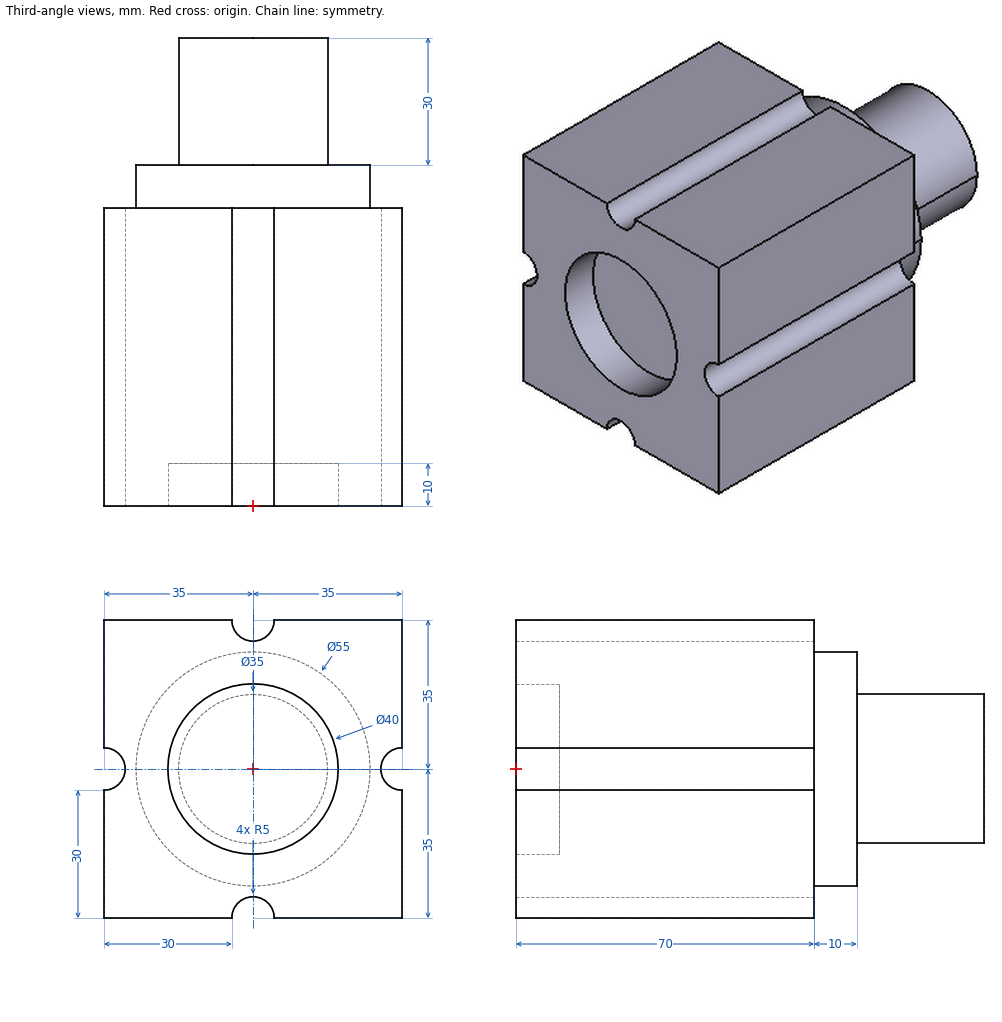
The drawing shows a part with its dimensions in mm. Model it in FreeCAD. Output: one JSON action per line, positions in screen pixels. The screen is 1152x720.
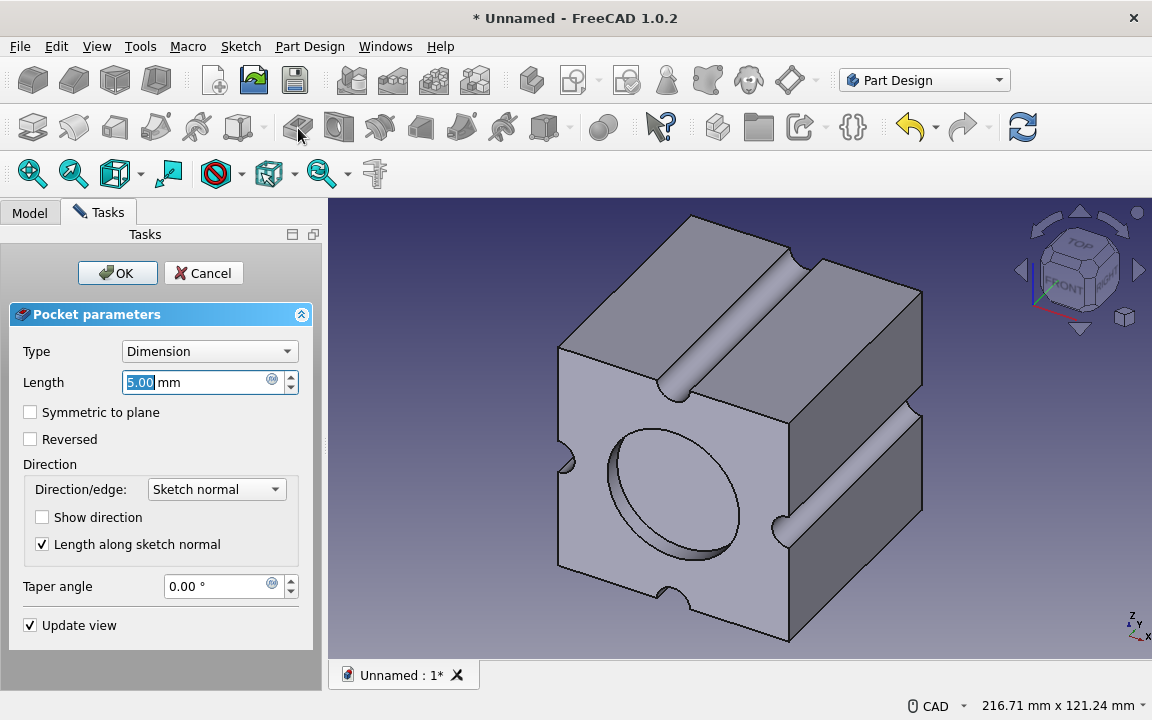
{"action": "type", "text": "10"}
{"action": "key", "text": "Tab"}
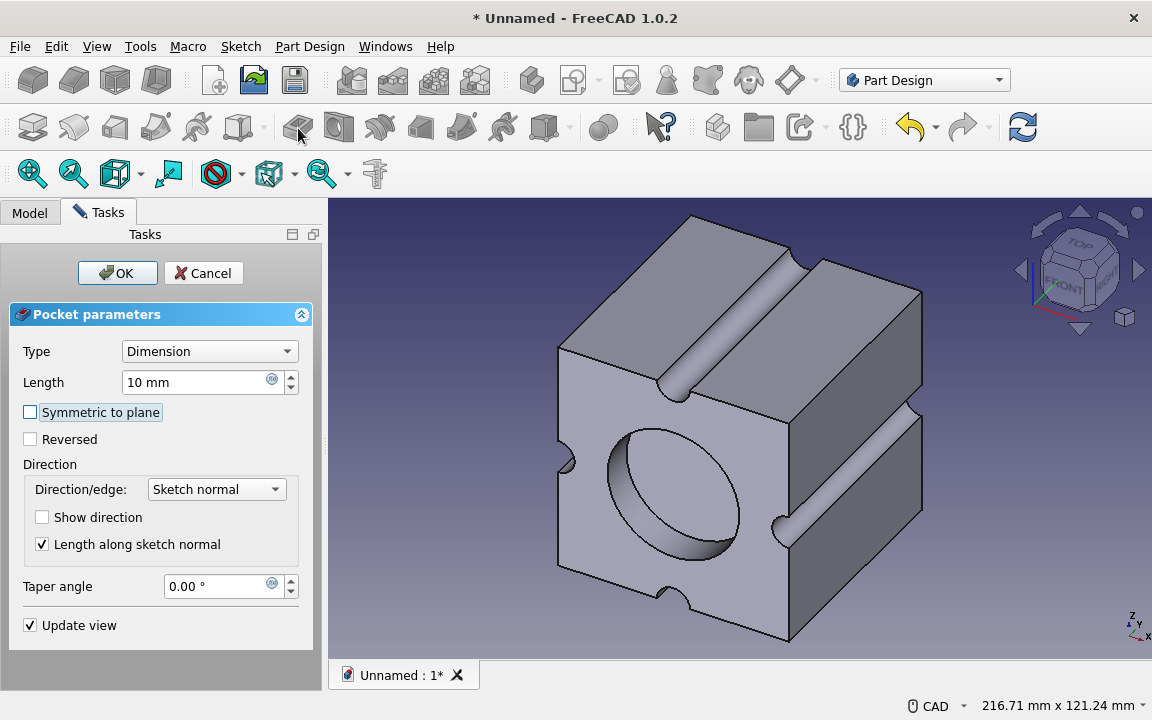
{"action": "left_click", "coordinate": [118, 273]}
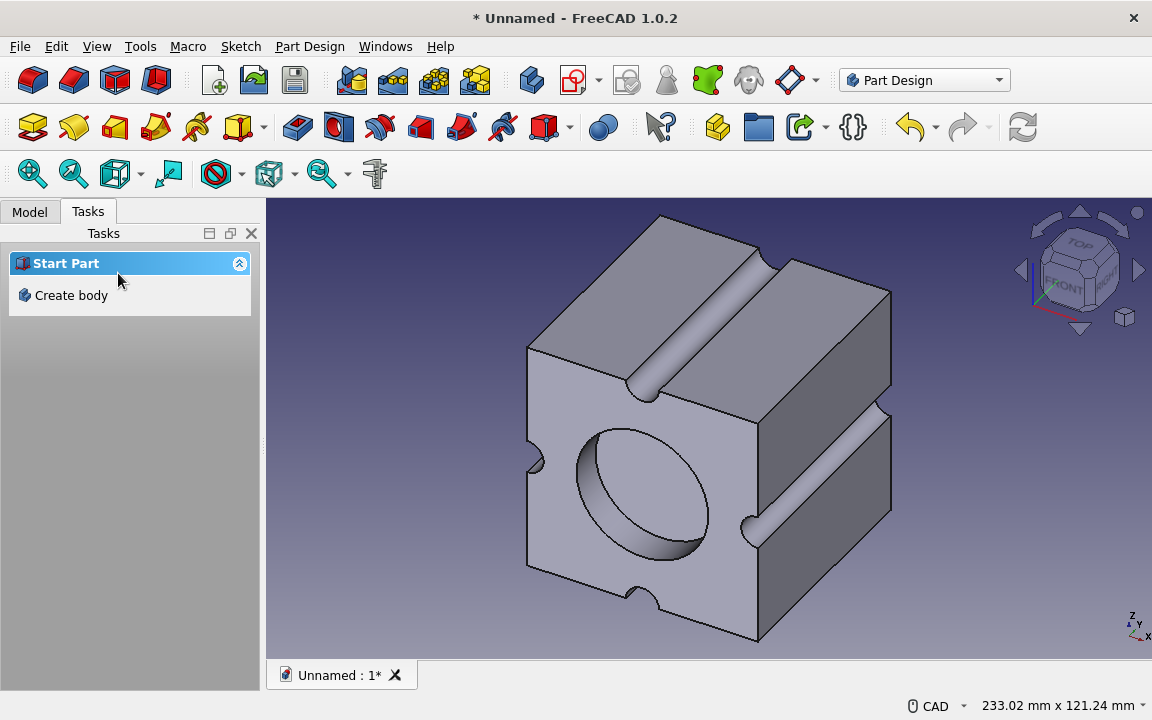
{"action": "key", "text": "4"}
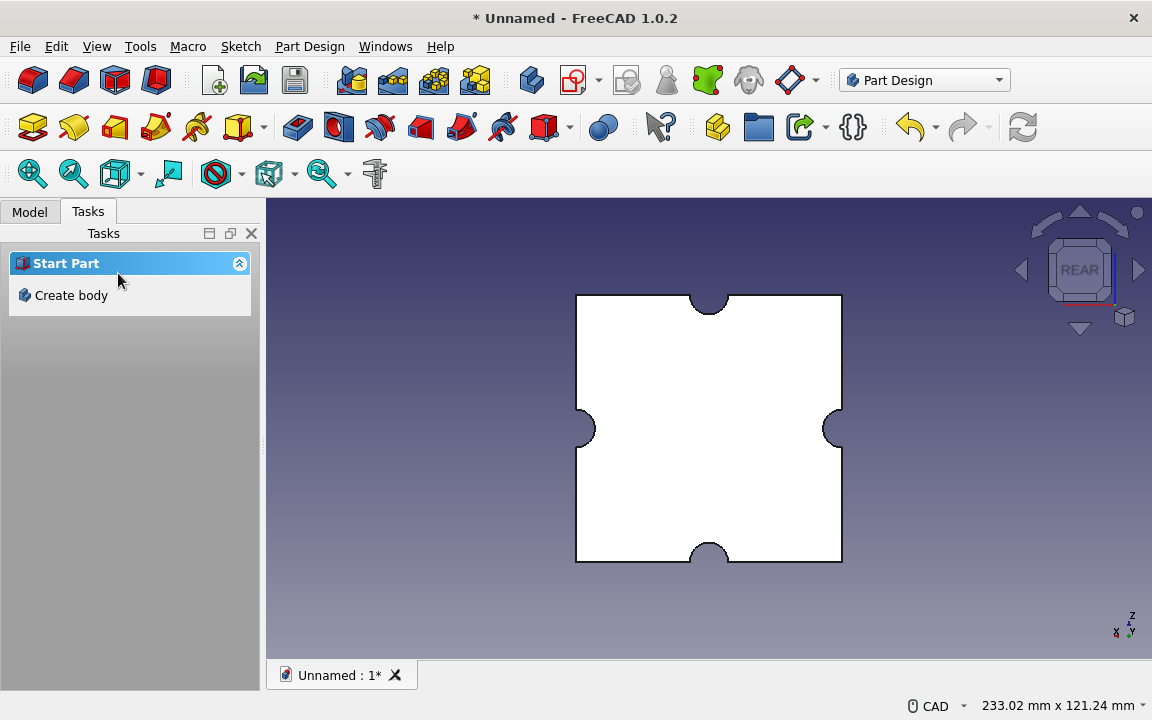
{"action": "left_click", "coordinate": [709, 428]}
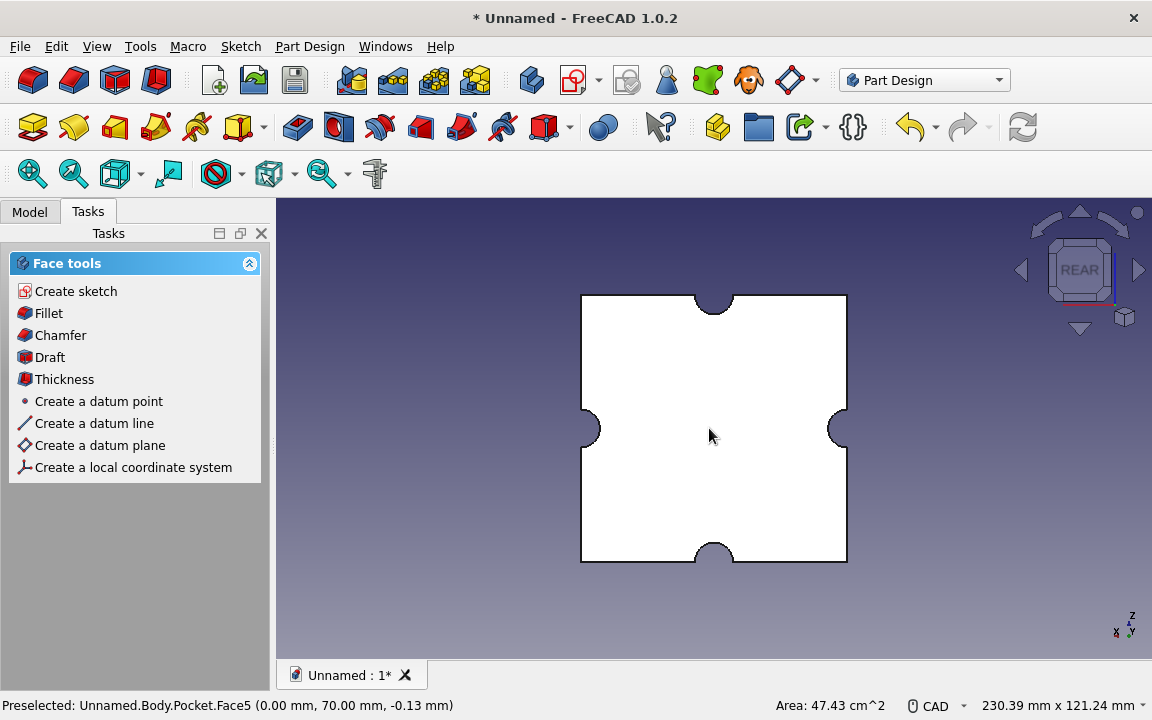
{"action": "left_click", "coordinate": [572, 80]}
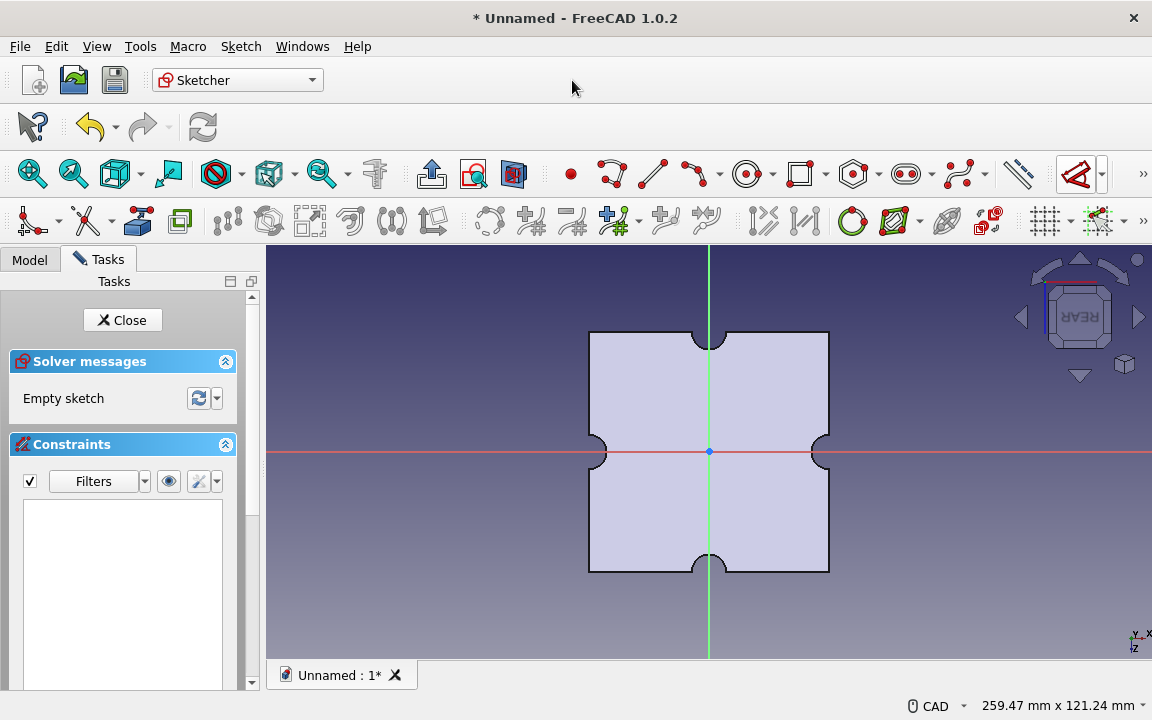
{"action": "left_click", "coordinate": [746, 174]}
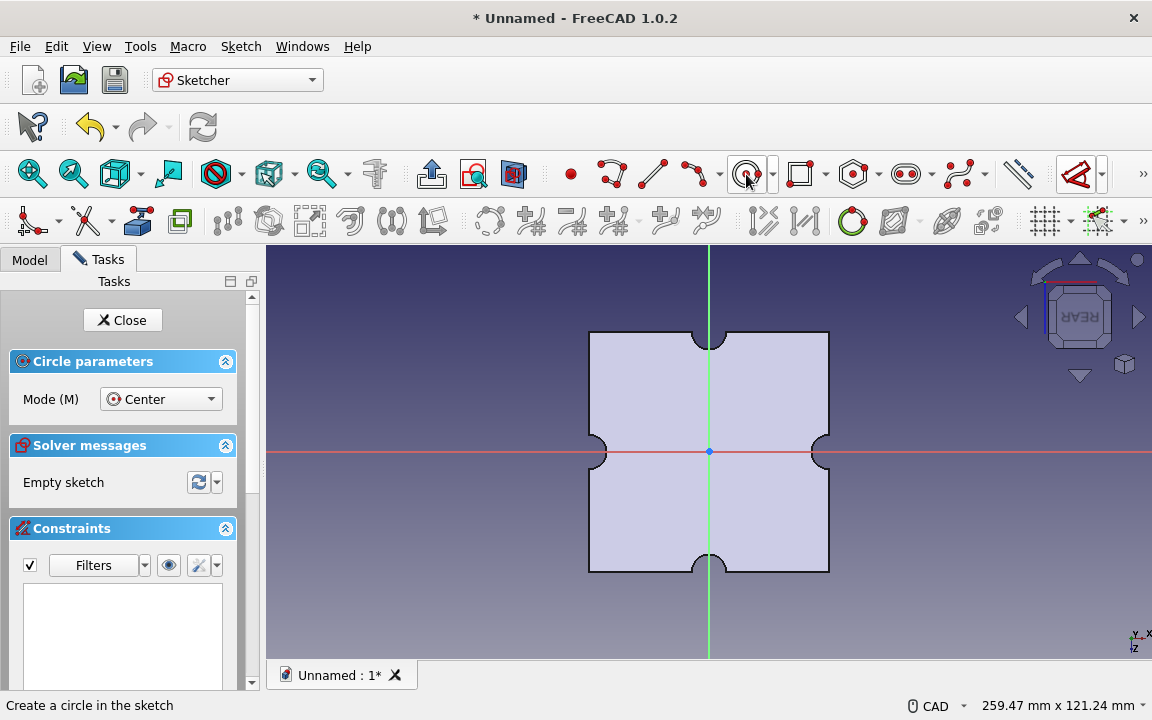
{"action": "left_click", "coordinate": [709, 452]}
{"action": "mouse_move", "coordinate": [775, 386]}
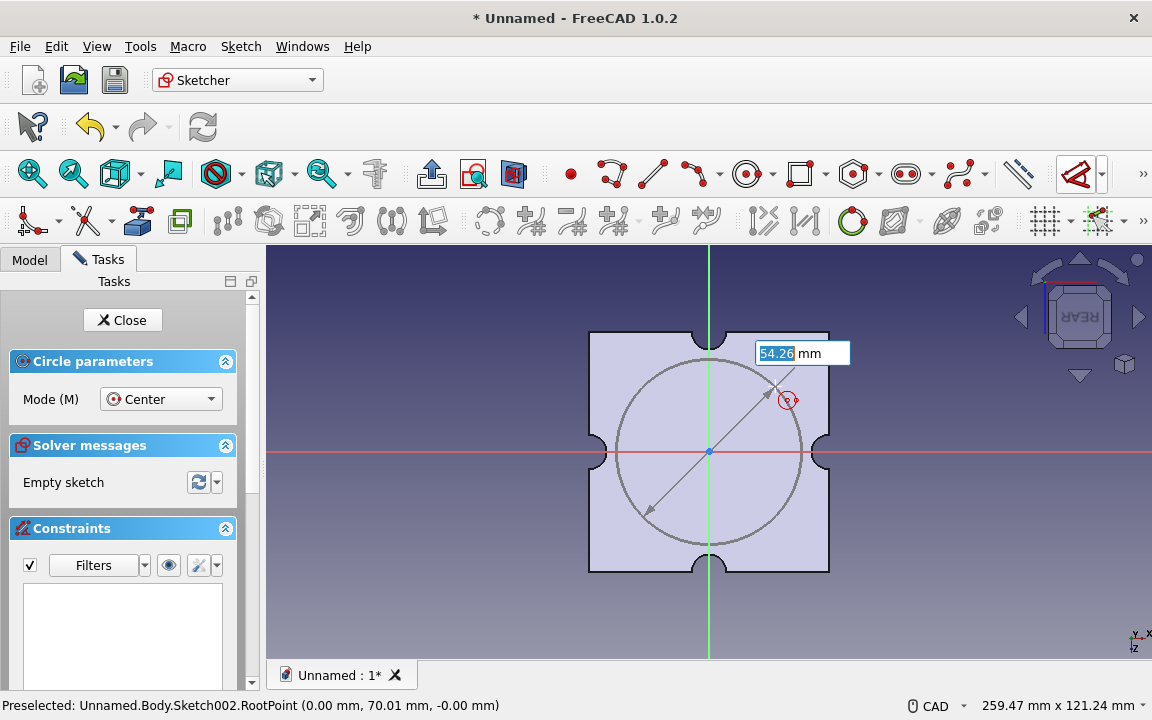
{"action": "type", "text": "55"}
{"action": "key", "text": "Return"}
{"action": "key", "text": "Escape"}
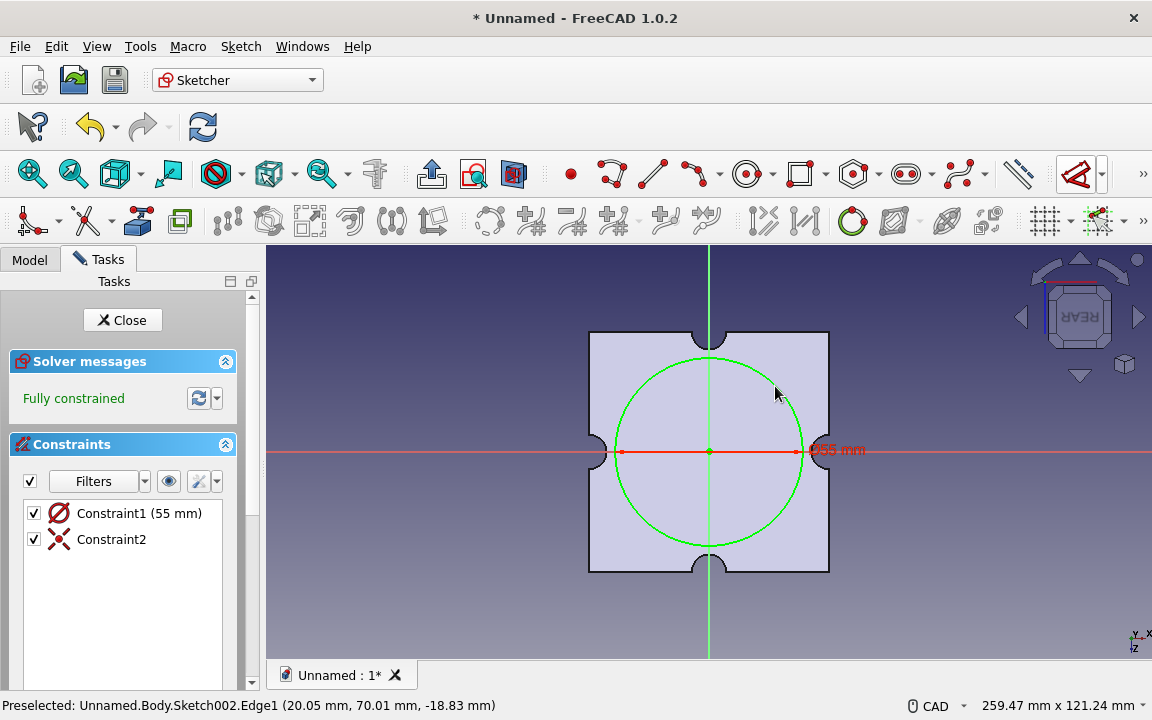
{"action": "left_click", "coordinate": [123, 320]}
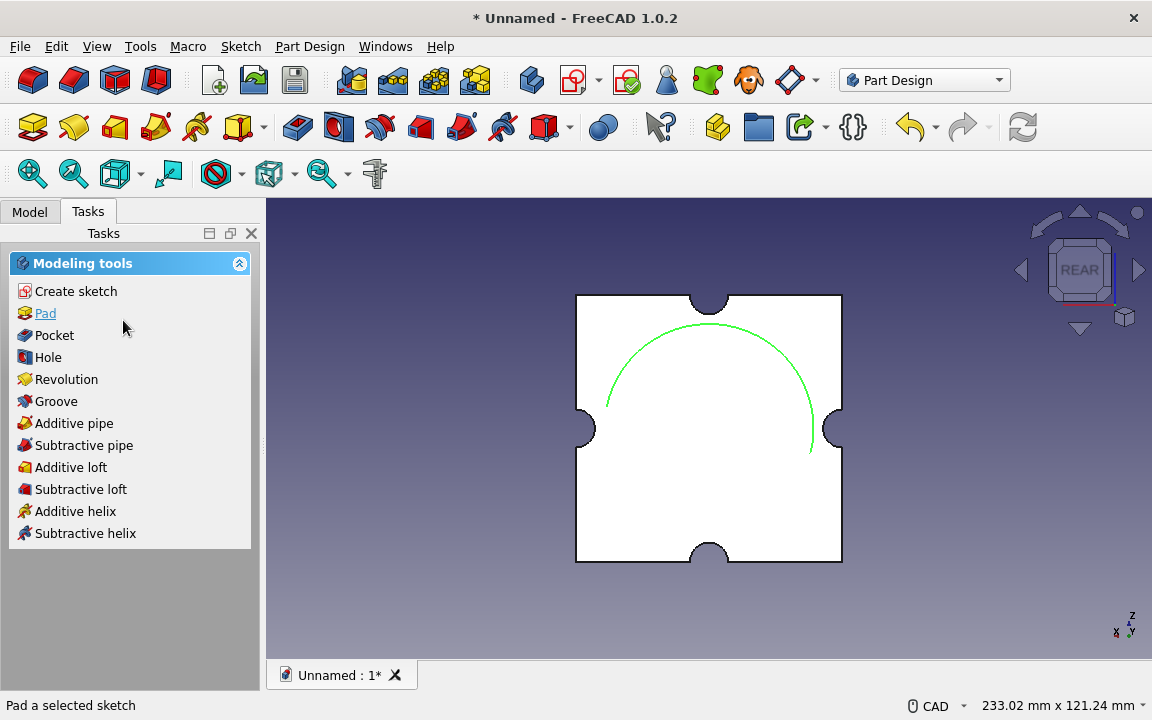
{"action": "left_click", "coordinate": [33, 128]}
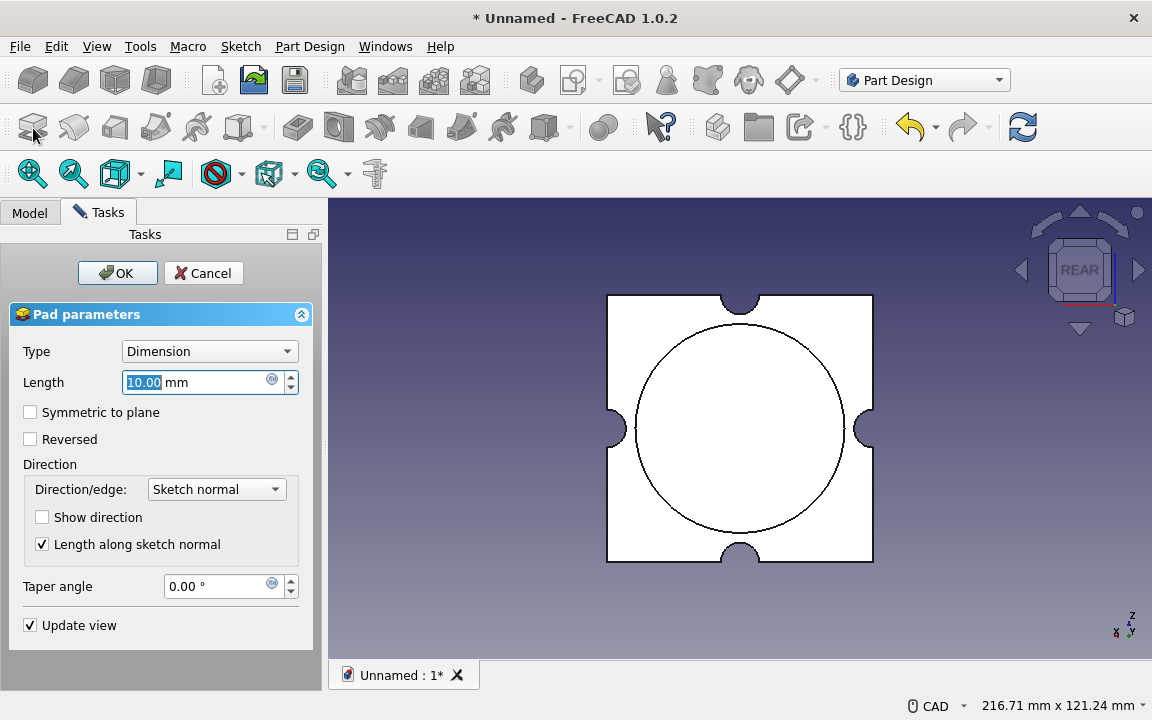
{"action": "type", "text": "10"}
{"action": "key", "text": "Tab"}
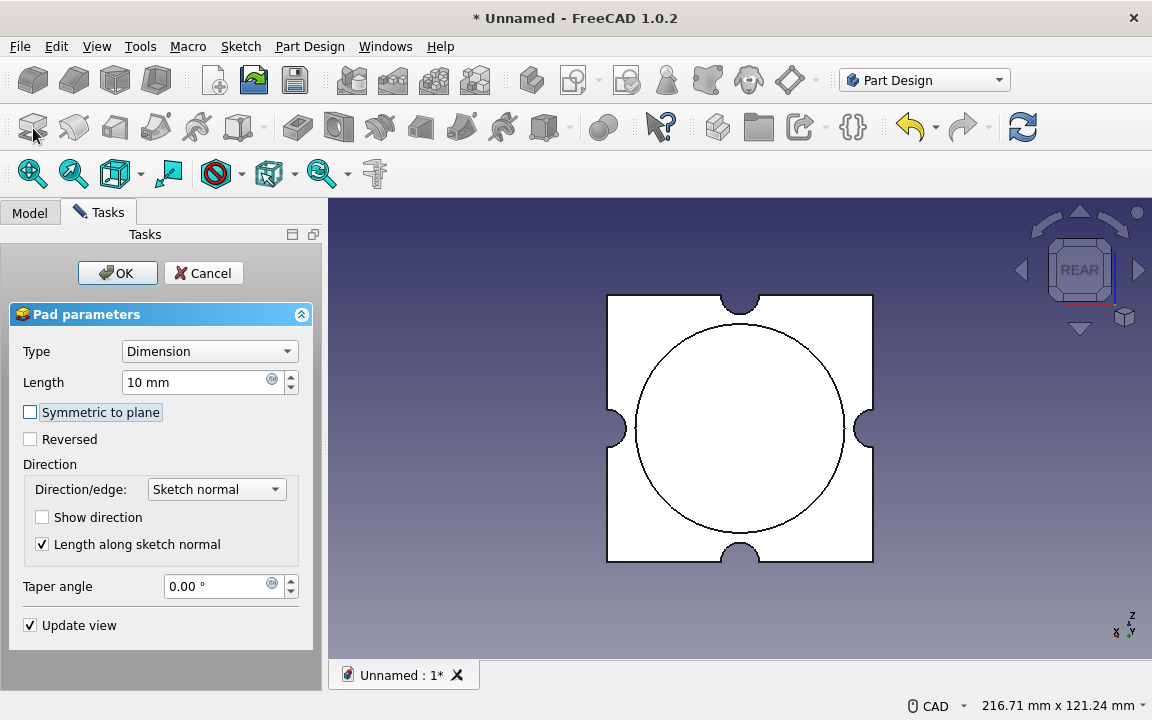
{"action": "left_click", "coordinate": [118, 273]}